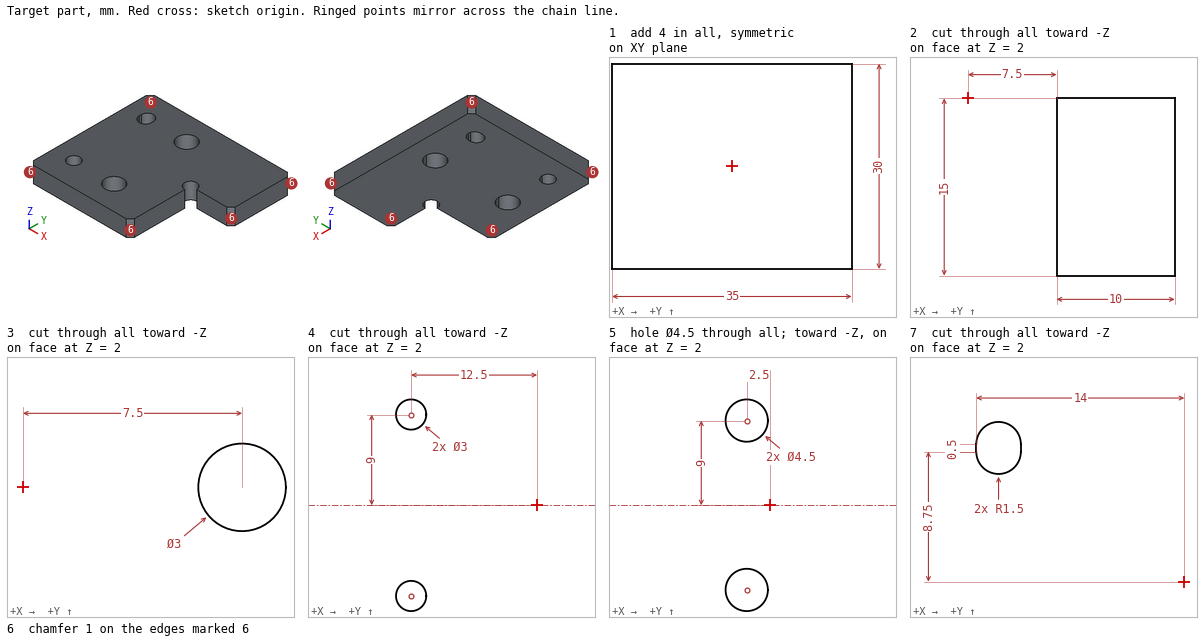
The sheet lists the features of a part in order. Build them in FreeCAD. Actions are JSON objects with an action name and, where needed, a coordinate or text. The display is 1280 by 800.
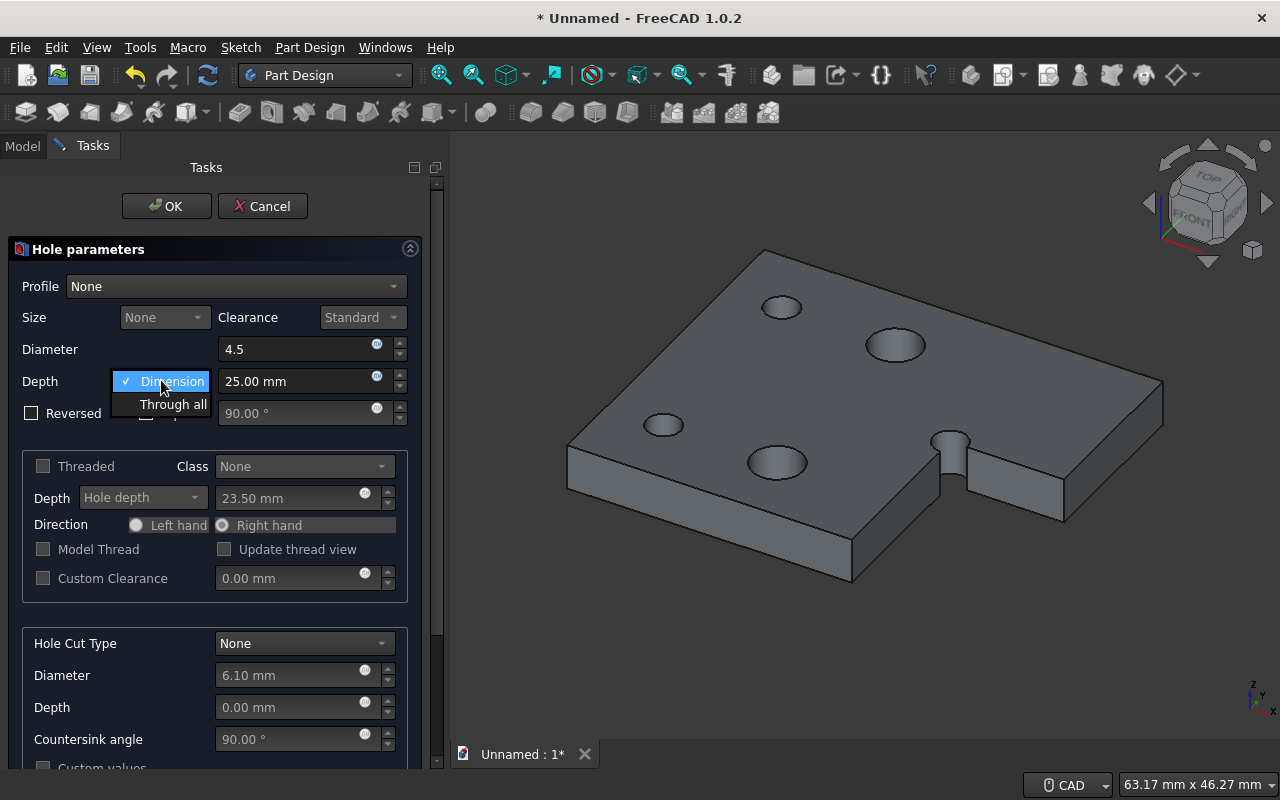
{"action": "left_click", "coordinate": [160, 404]}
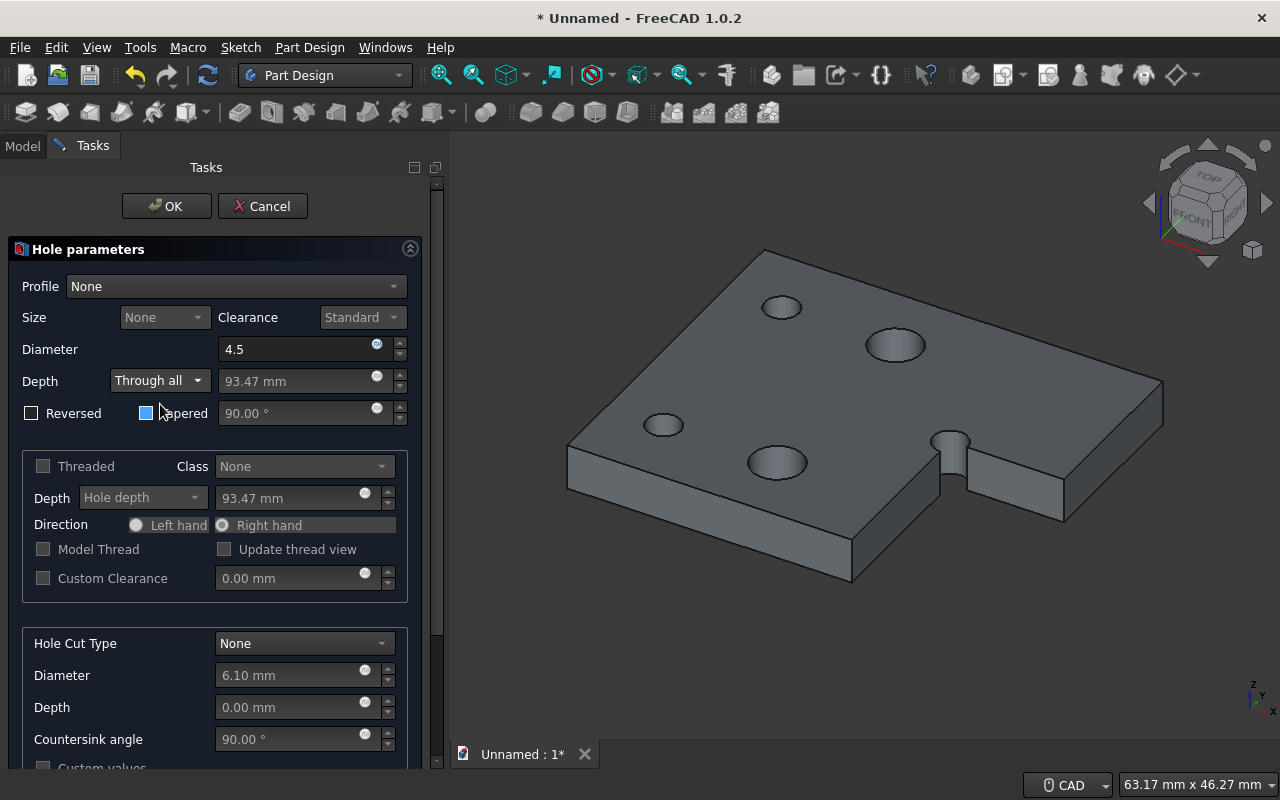
{"action": "left_click", "coordinate": [167, 206]}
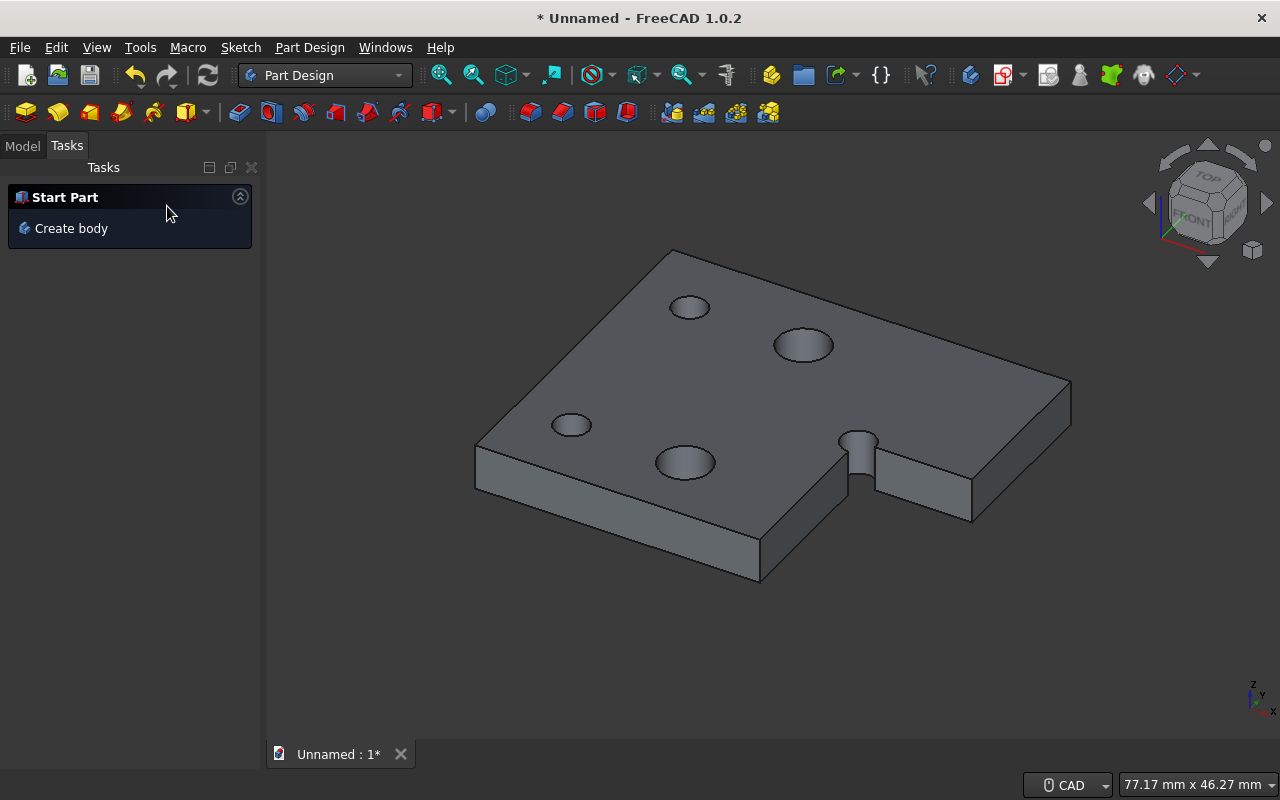
{"action": "left_click", "coordinate": [972, 500]}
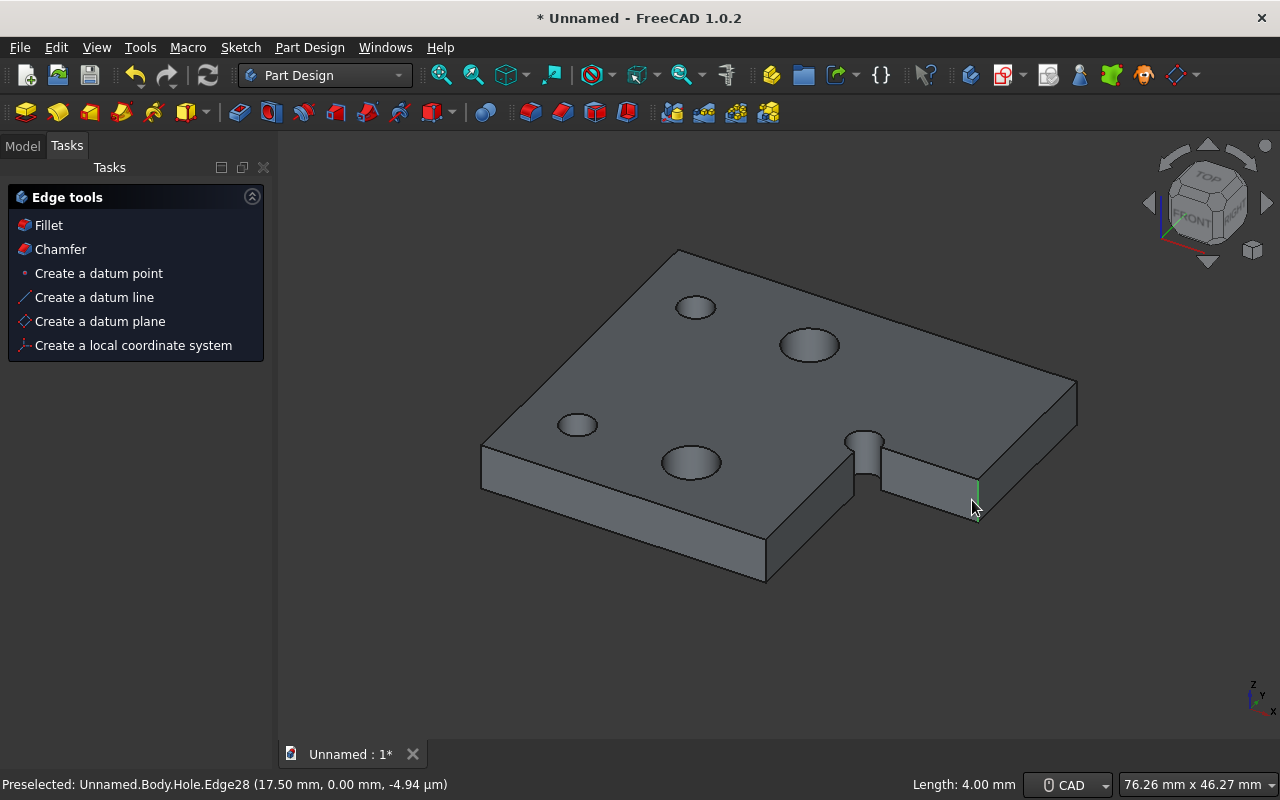
{"action": "left_click", "coordinate": [766, 560], "text": "ctrl"}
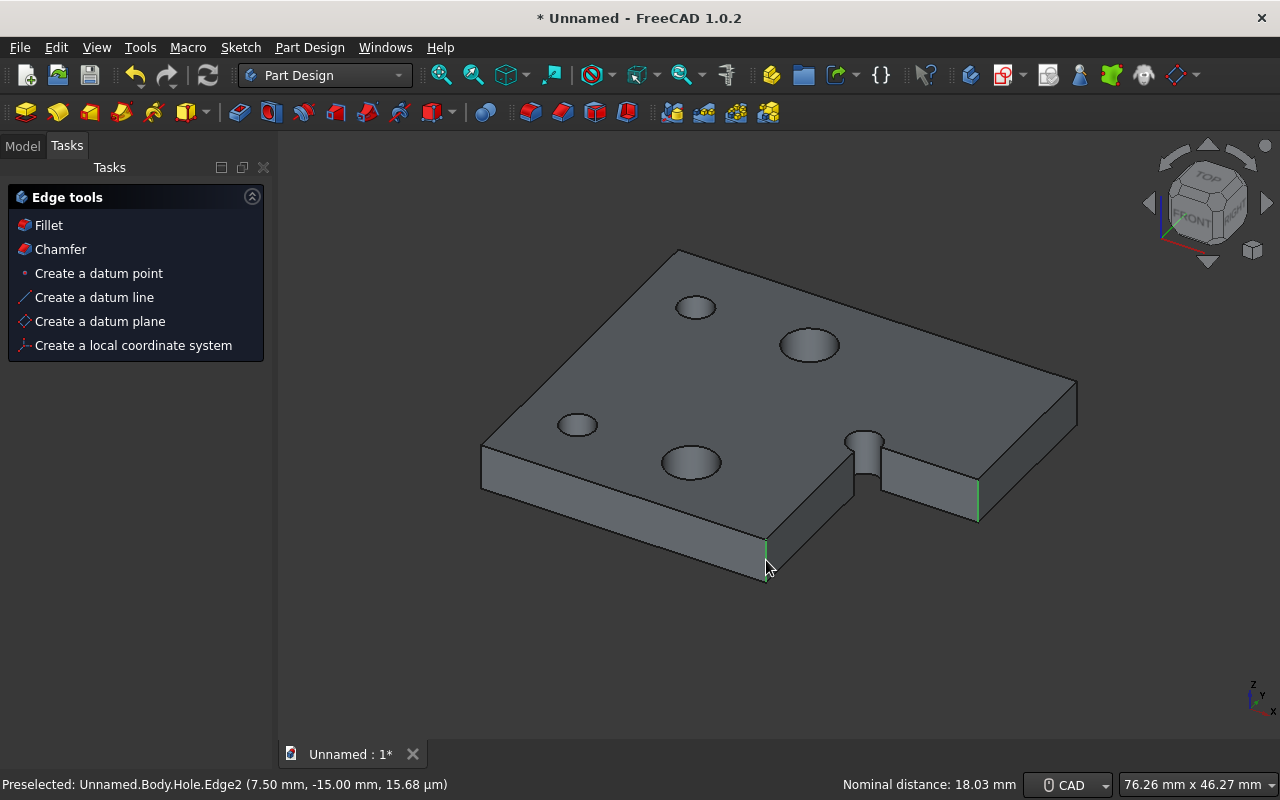
{"action": "key", "text": "0"}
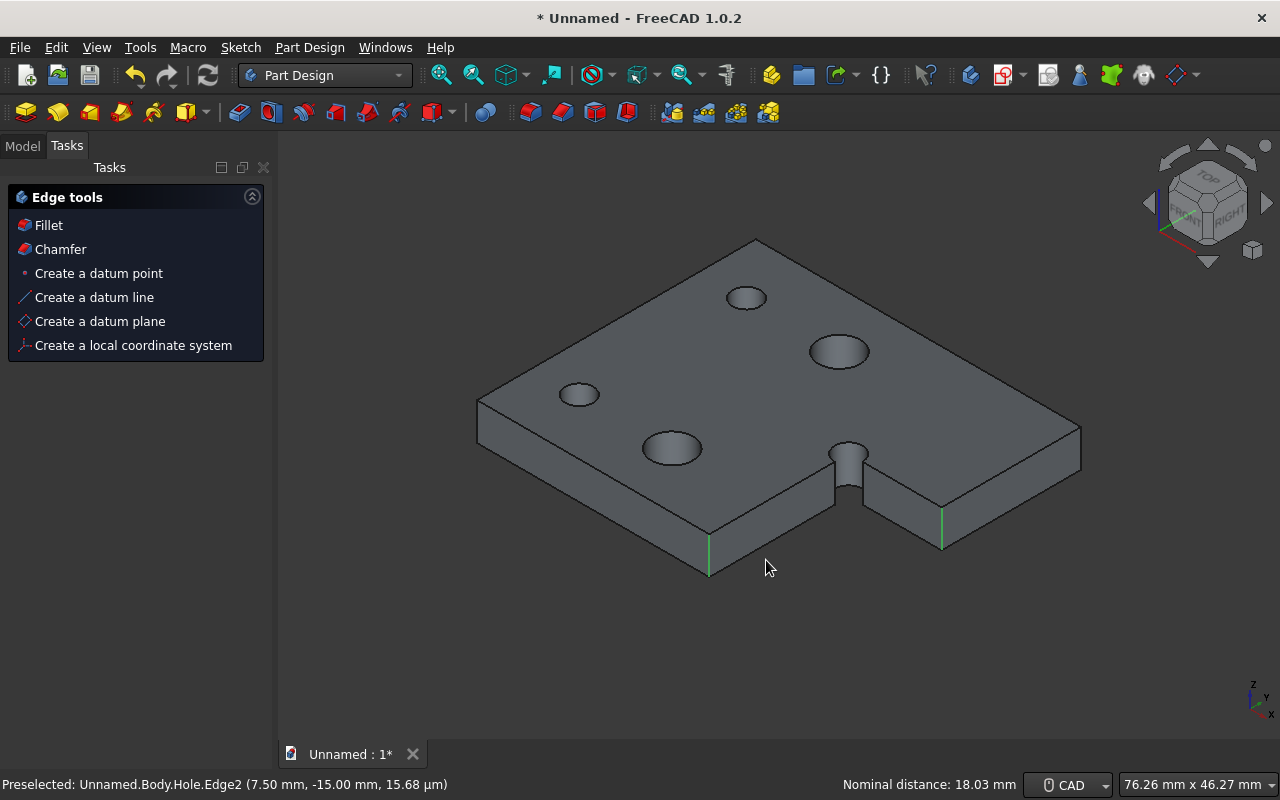
{"action": "key", "text": "2"}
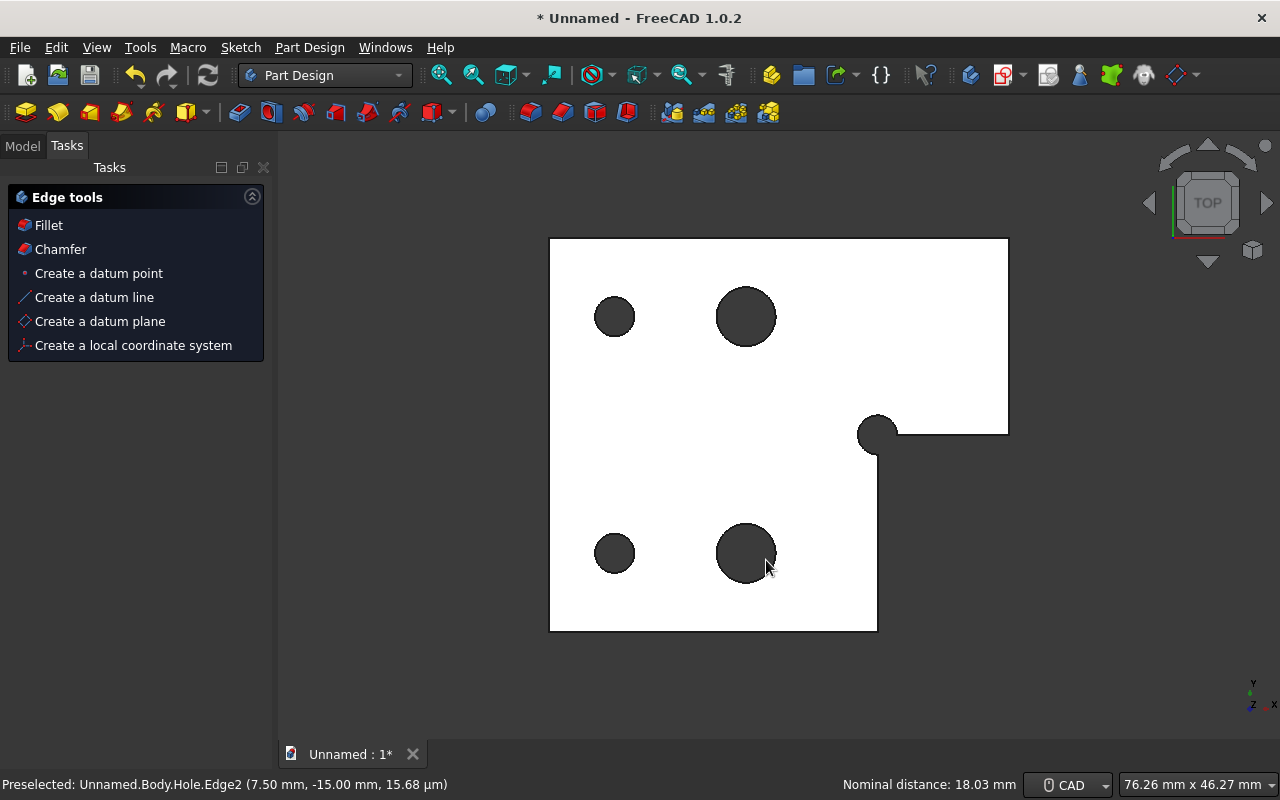
{"action": "key", "text": "1"}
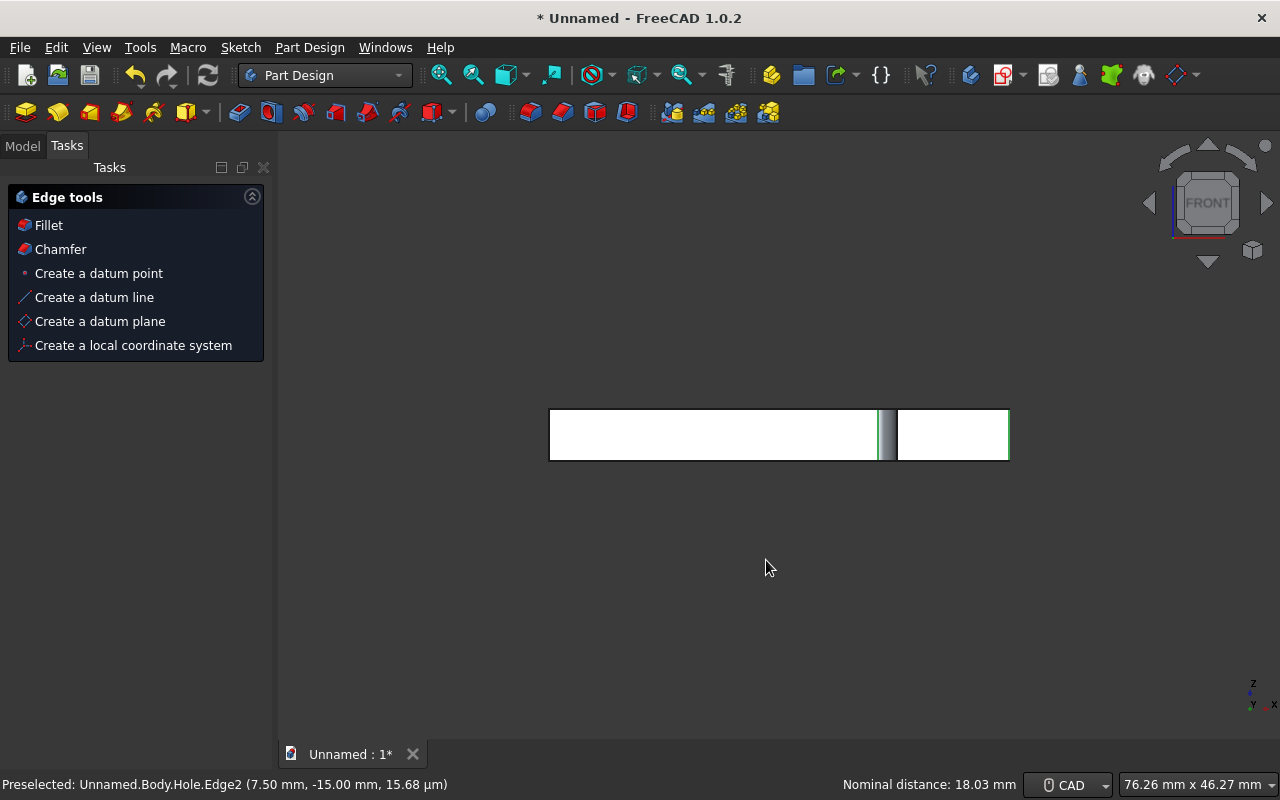
{"action": "left_click", "coordinate": [549, 434], "text": "ctrl"}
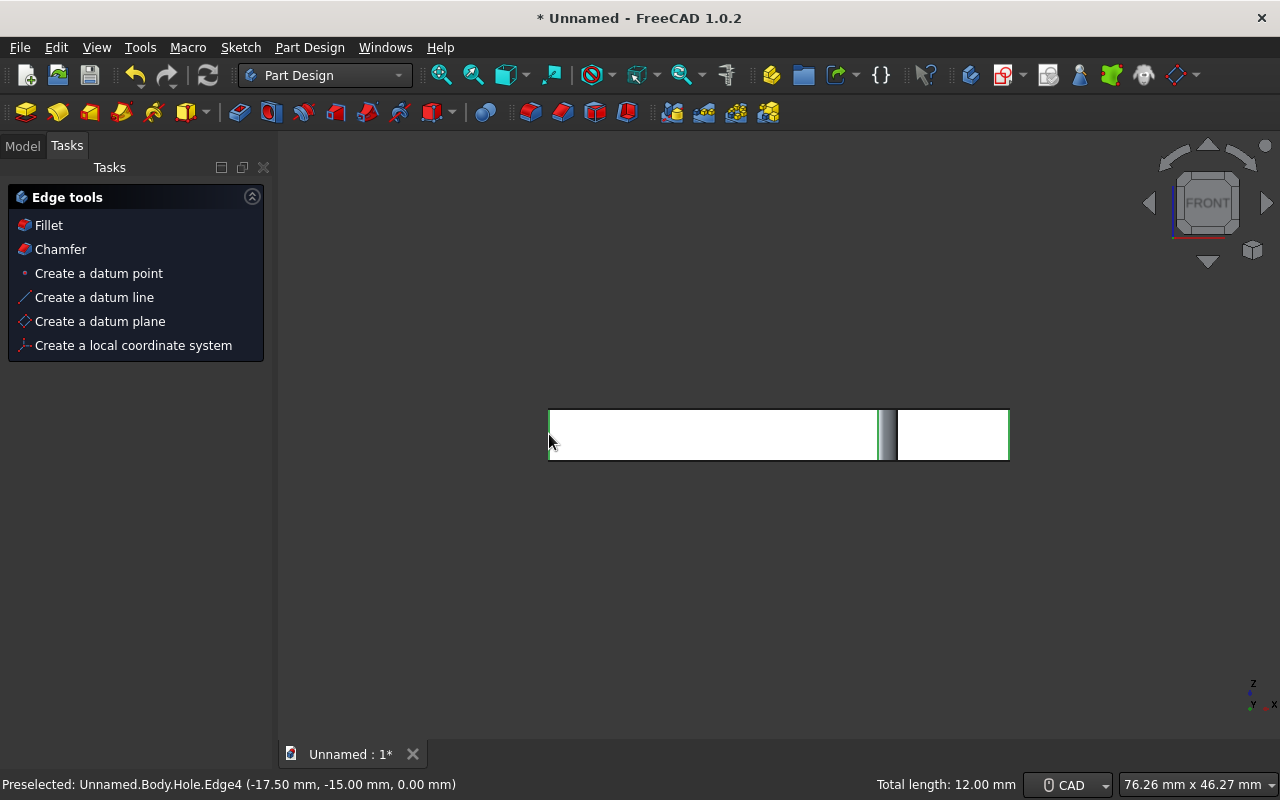
{"action": "key", "text": "3"}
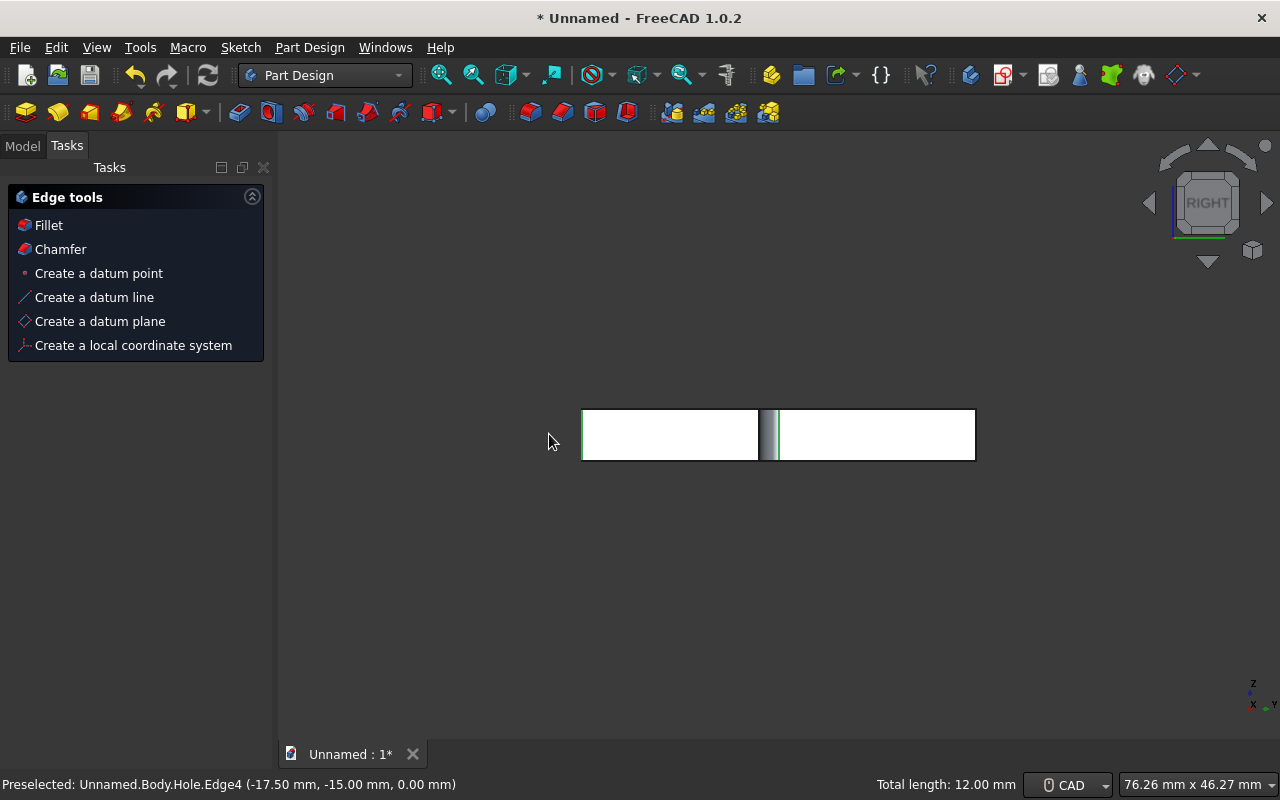
{"action": "key", "text": "v f"}